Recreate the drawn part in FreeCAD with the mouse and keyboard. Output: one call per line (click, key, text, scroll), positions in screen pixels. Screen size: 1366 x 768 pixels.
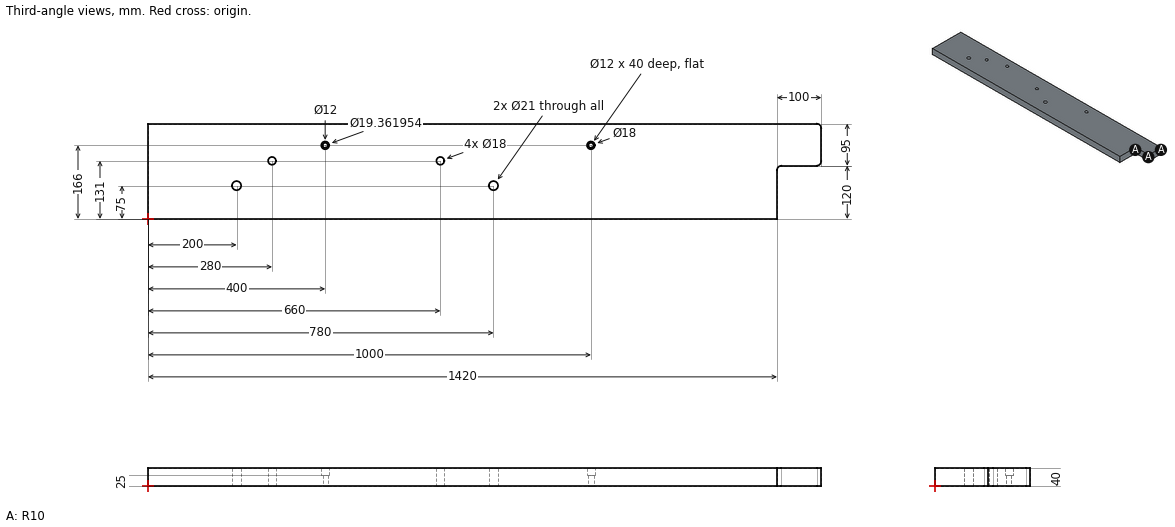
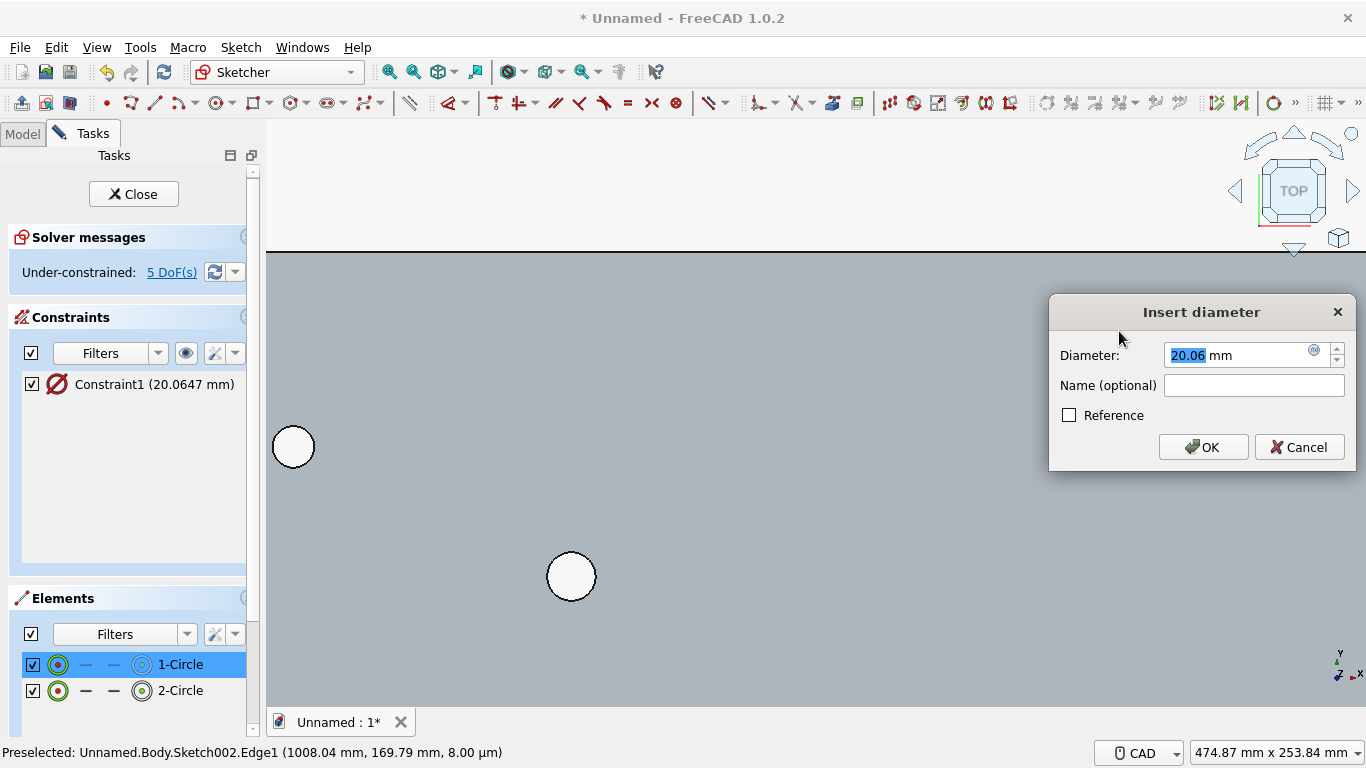
text(18)
key(Return)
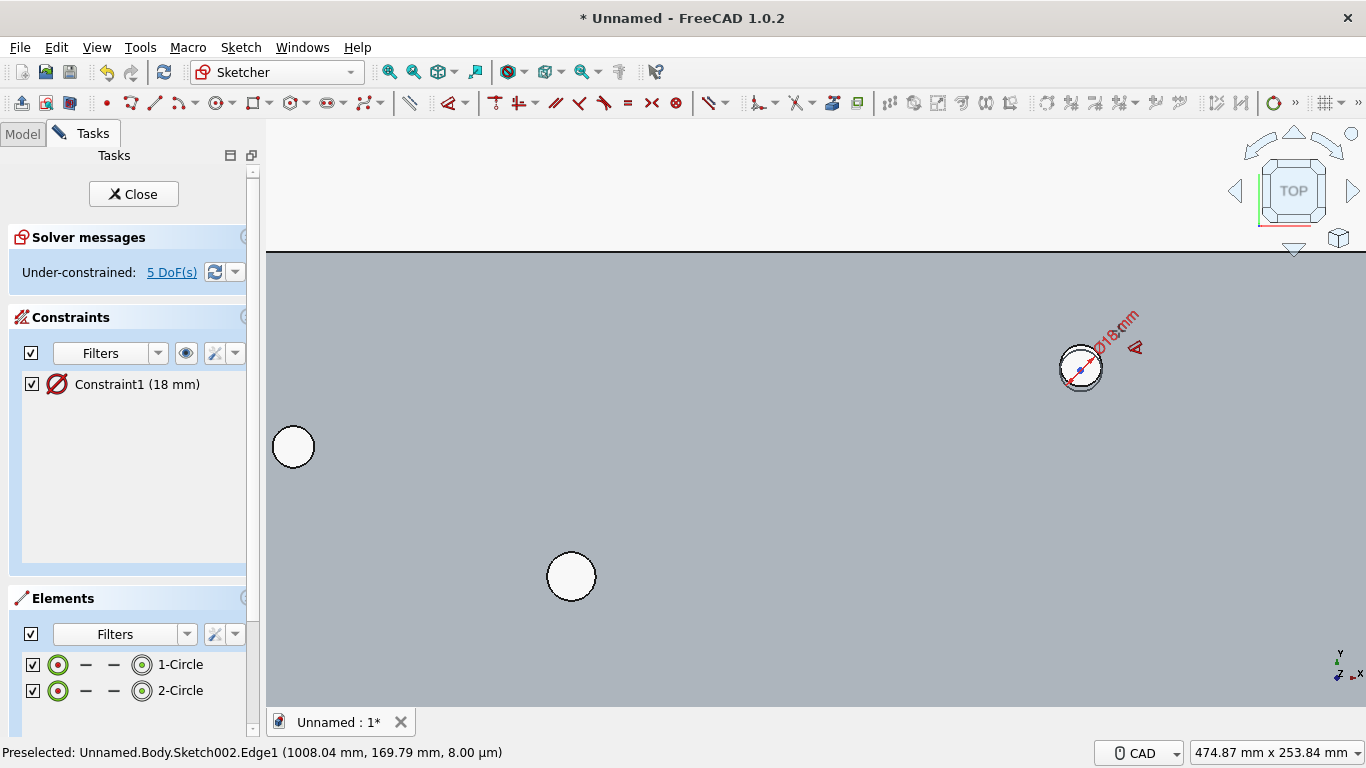
scroll(1098, 355, down, 6)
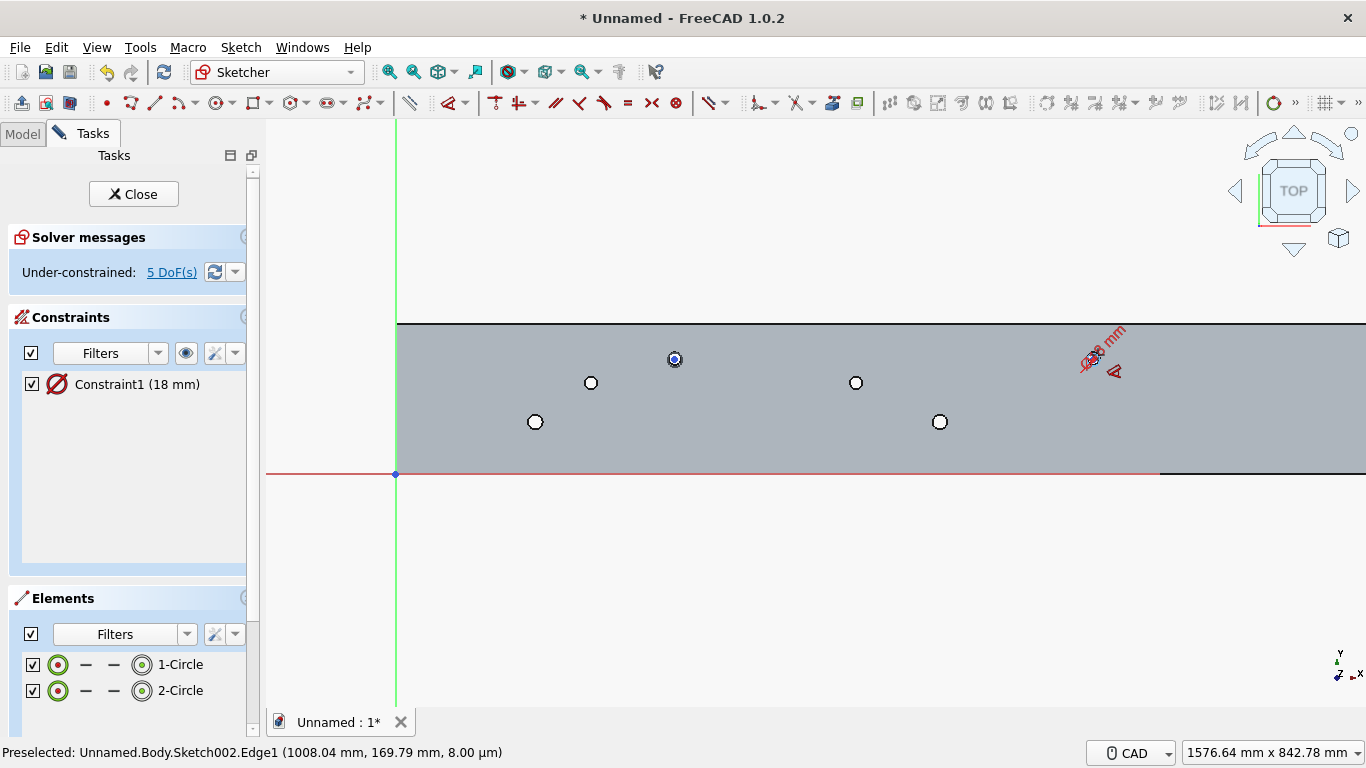
scroll(680, 355, up, 6)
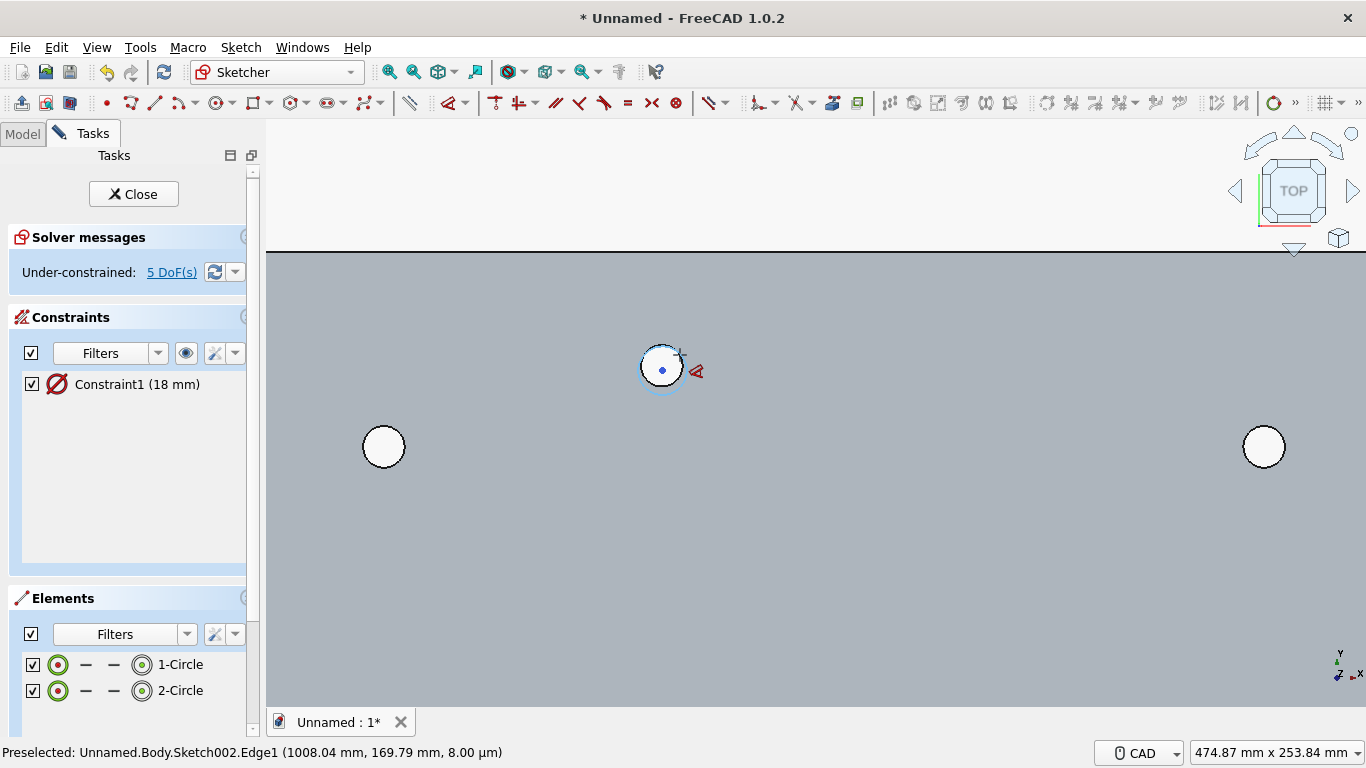
click(680, 353)
click(703, 330)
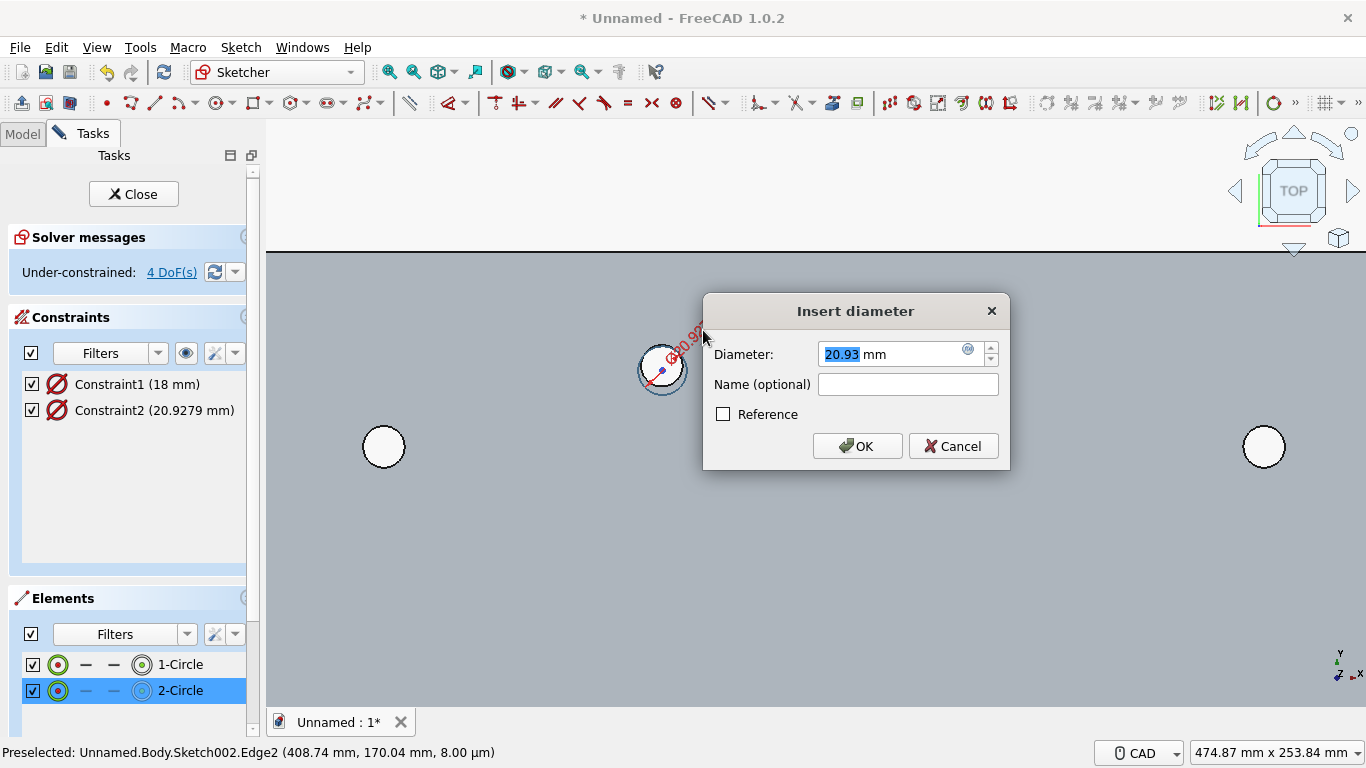
text(19.361954)
key(Return)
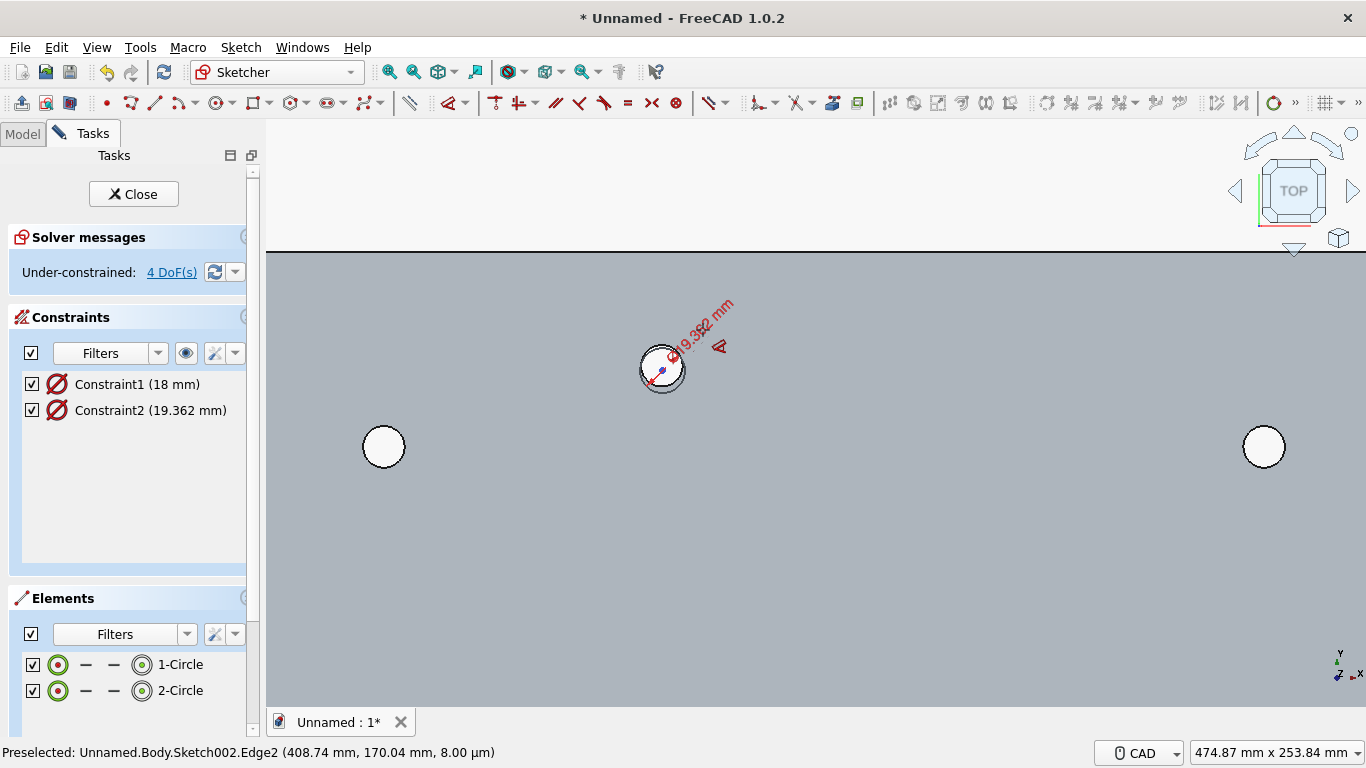
scroll(680, 355, down, 6)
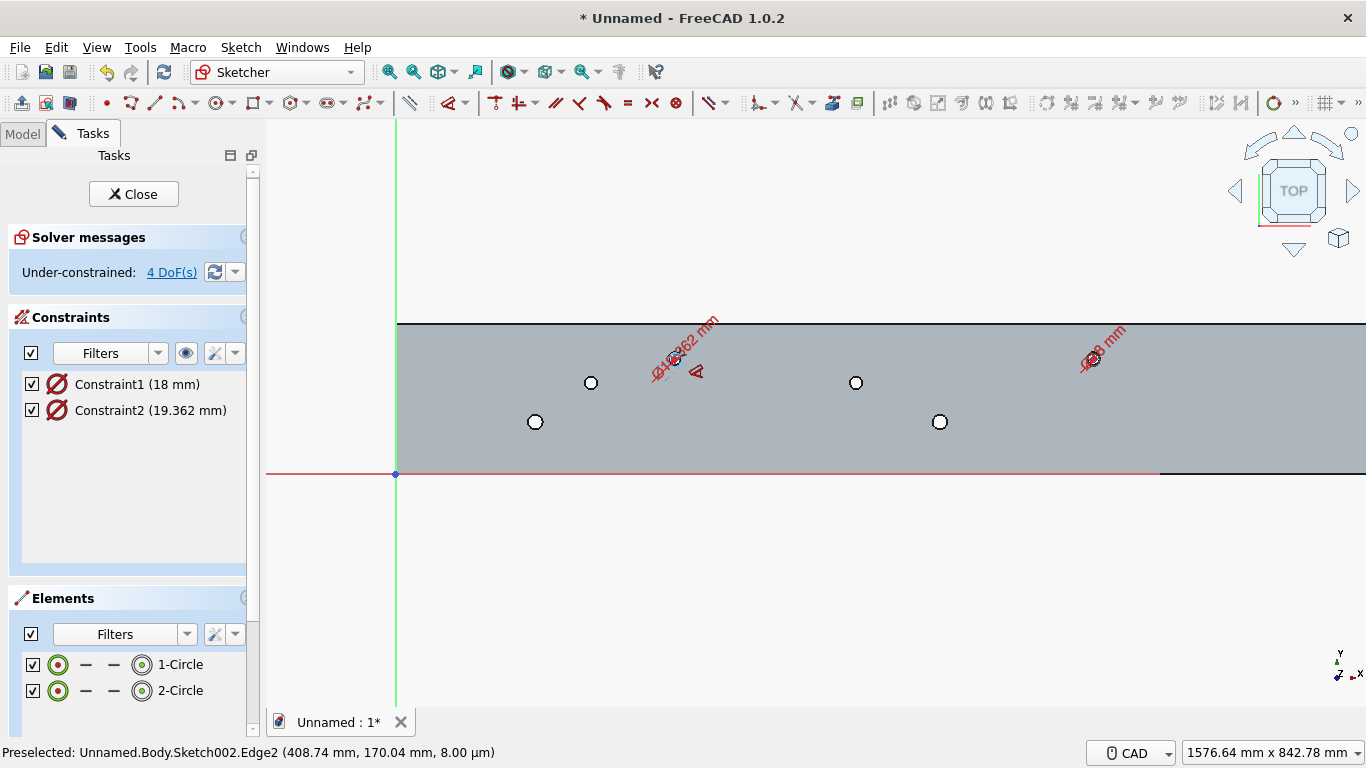
click(1093, 360)
click(362, 417)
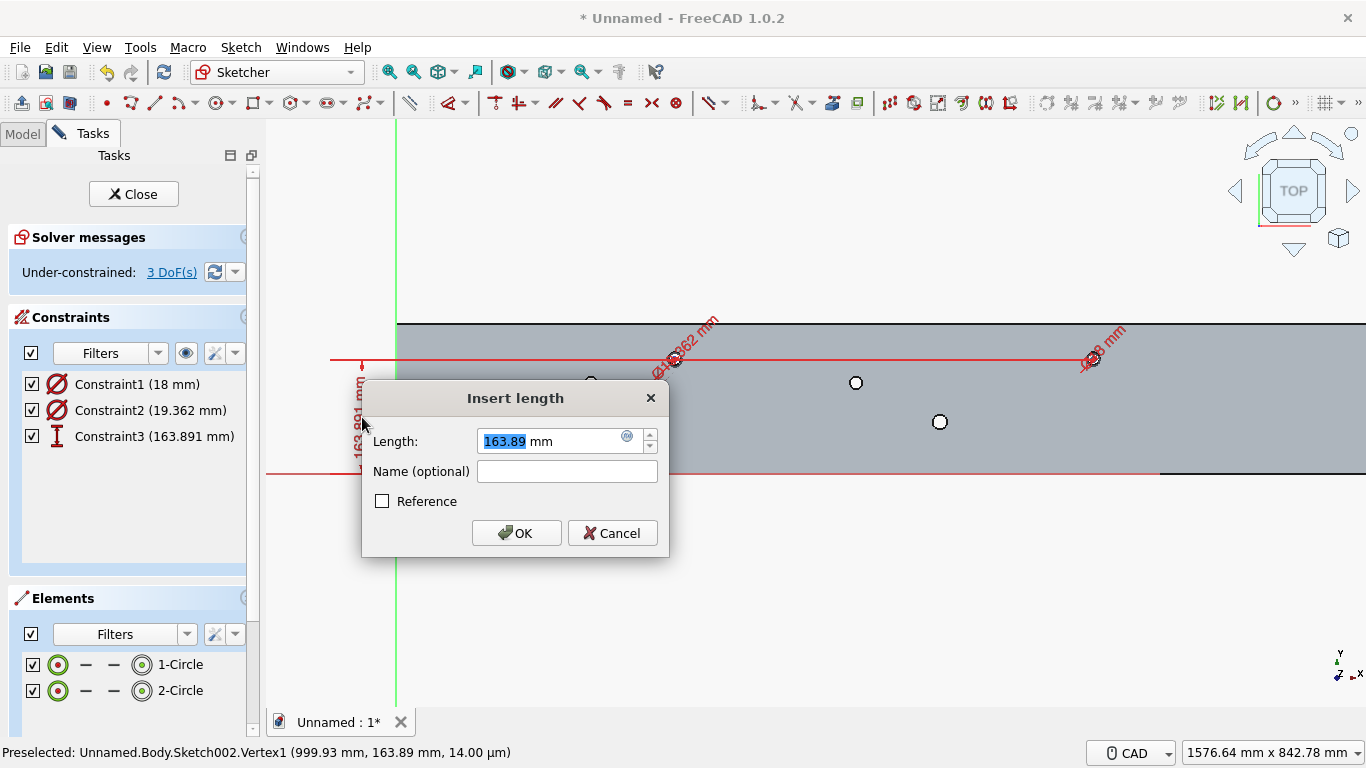
text(166)
key(Return)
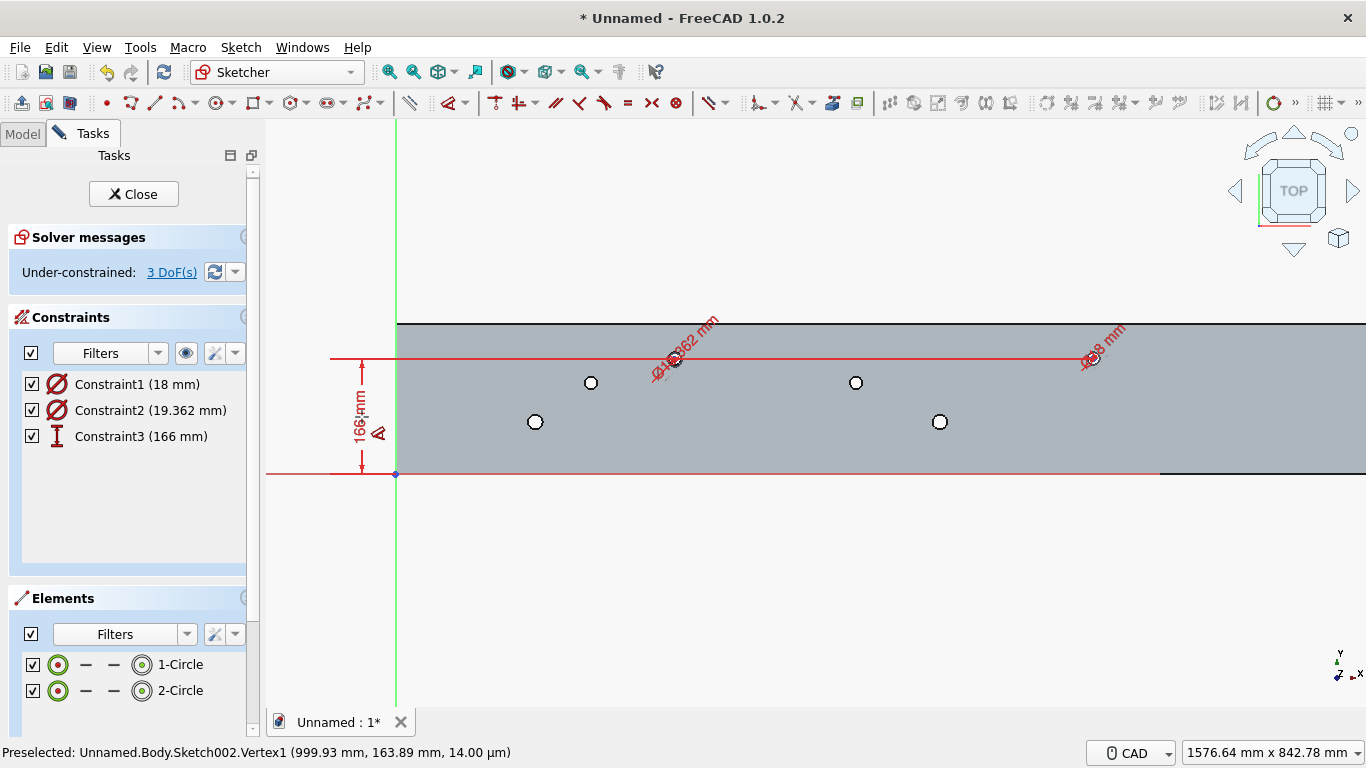
click(675, 360)
click(535, 508)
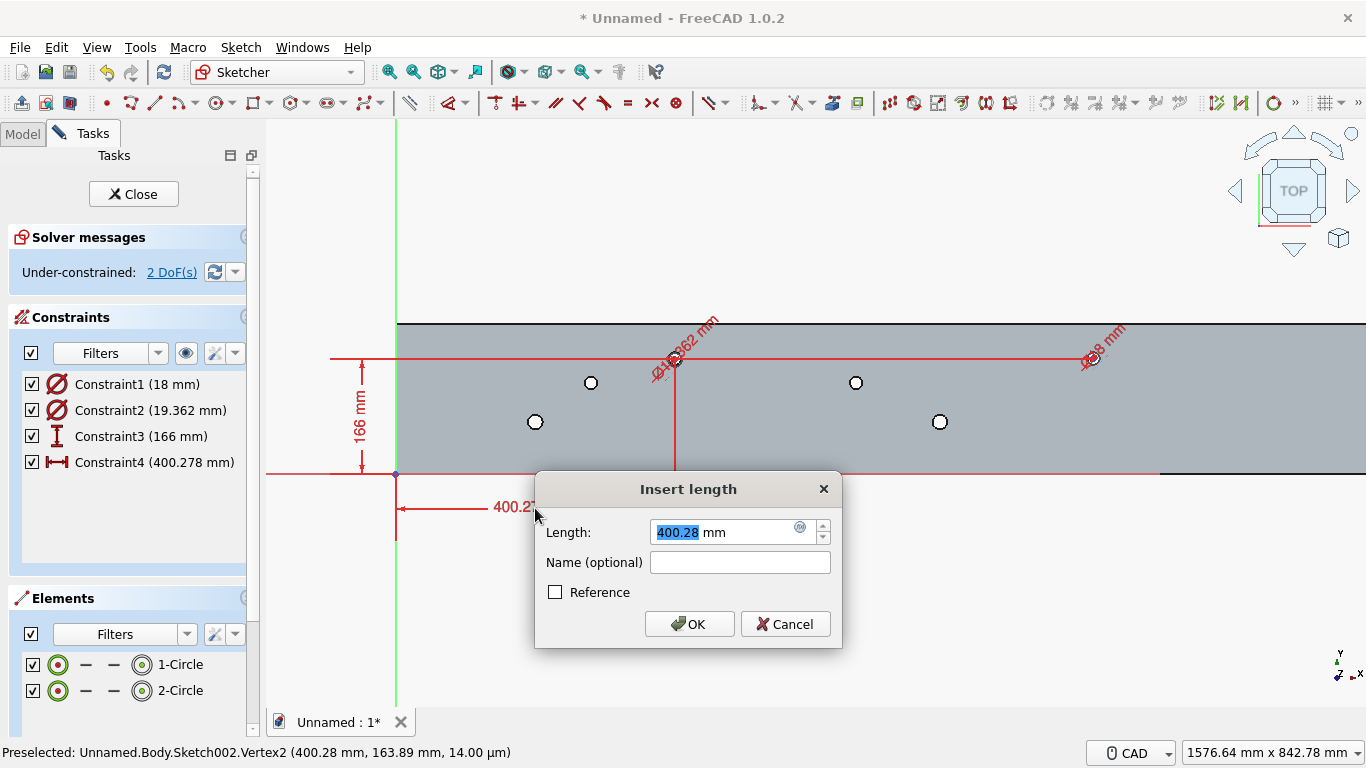
text(400)
key(Return)